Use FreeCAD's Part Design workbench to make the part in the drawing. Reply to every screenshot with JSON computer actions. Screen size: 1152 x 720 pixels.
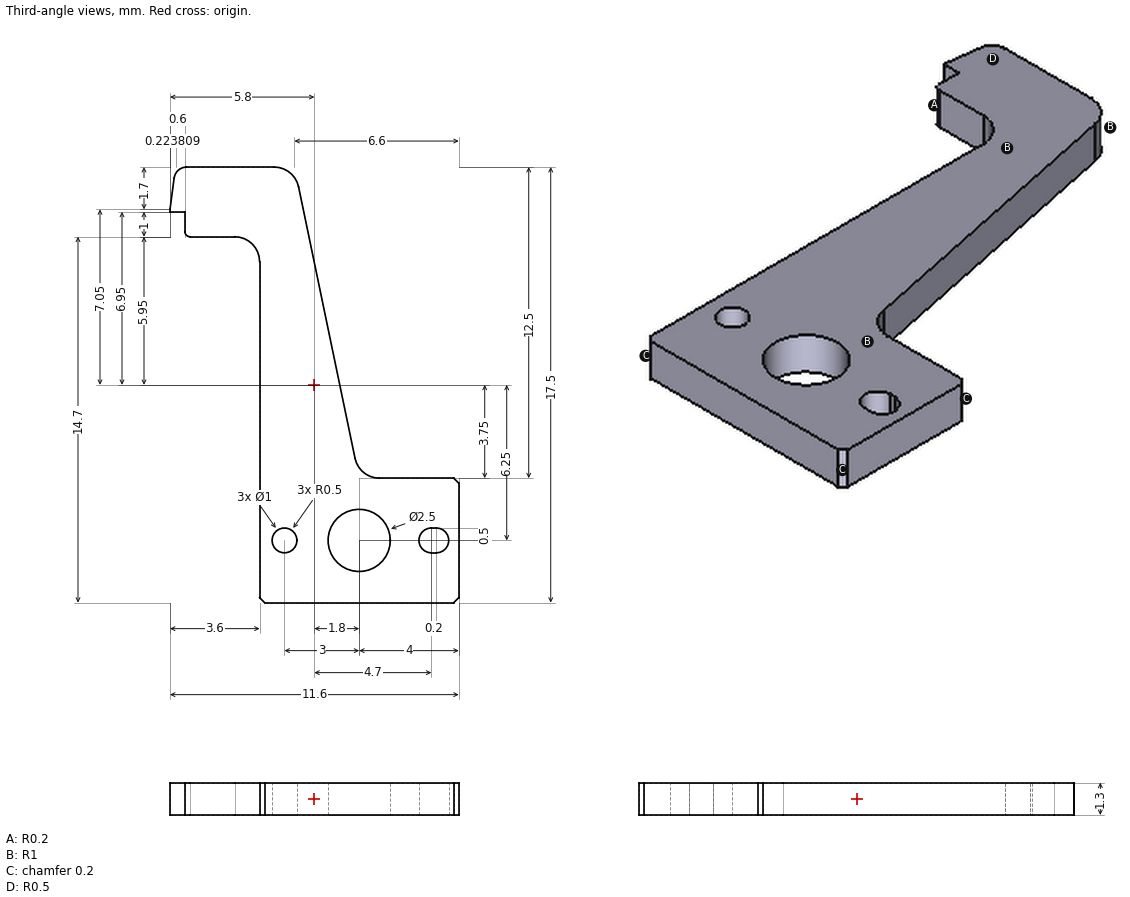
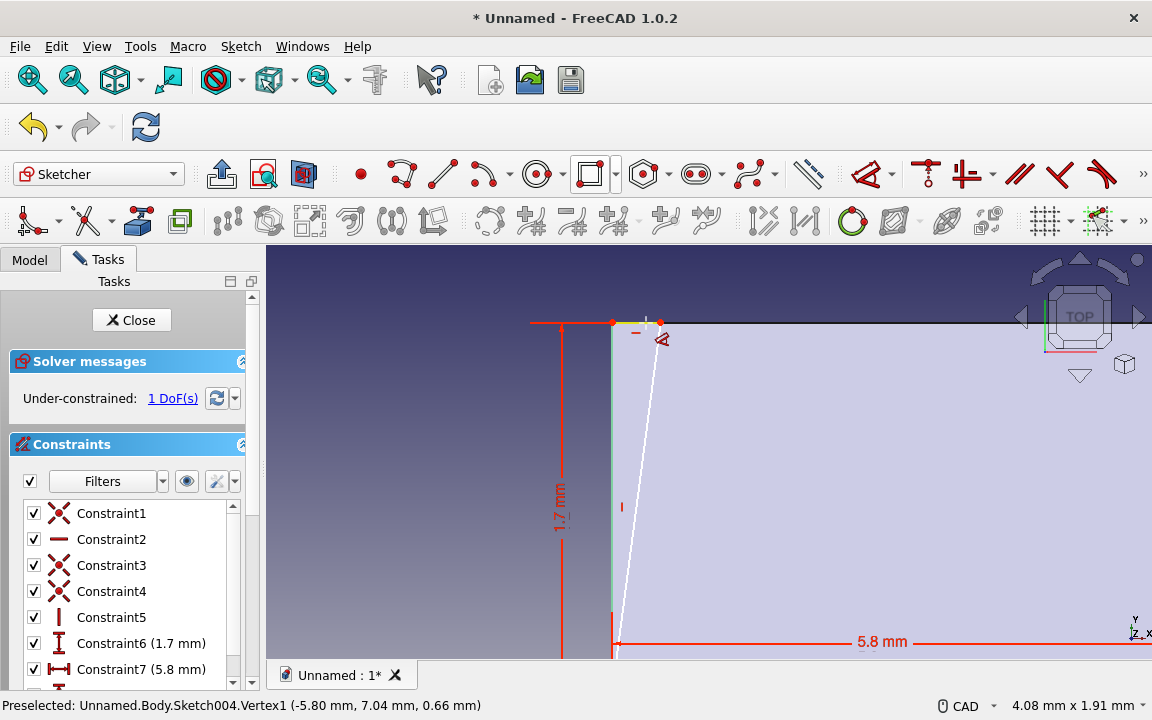
{"action": "left_click", "coordinate": [646, 323]}
{"action": "left_click", "coordinate": [636, 289]}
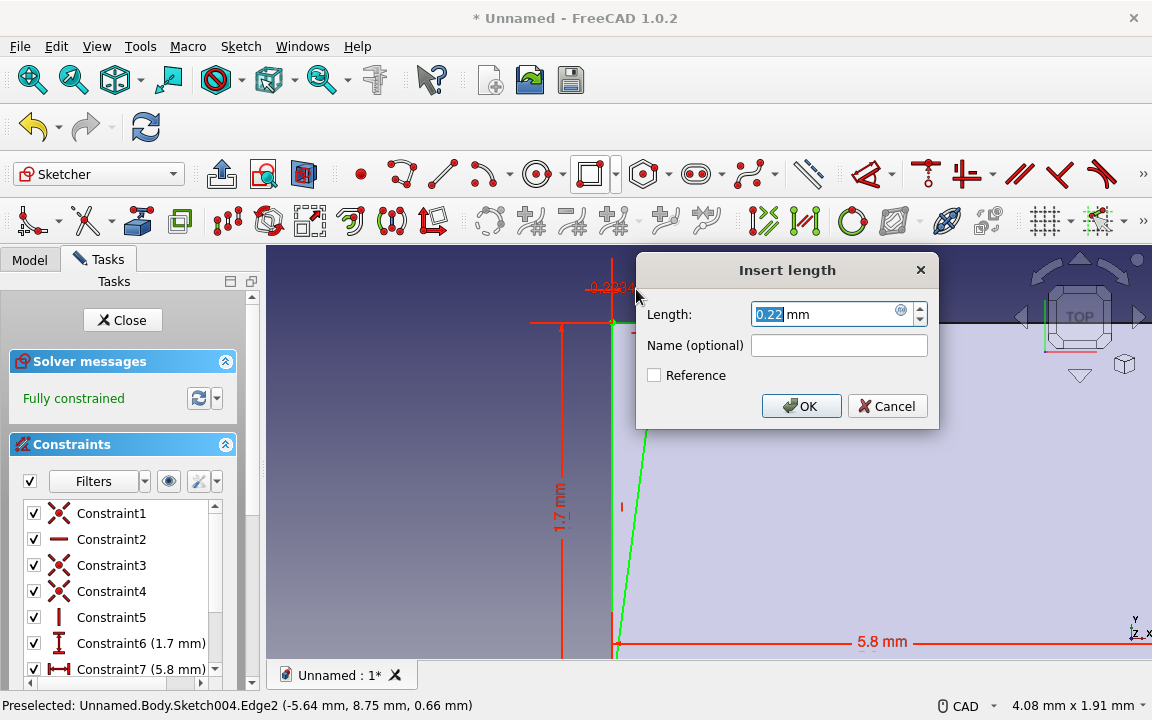
{"action": "type", "text": "0.223809"}
{"action": "key", "text": "Return"}
{"action": "key", "text": "Escape"}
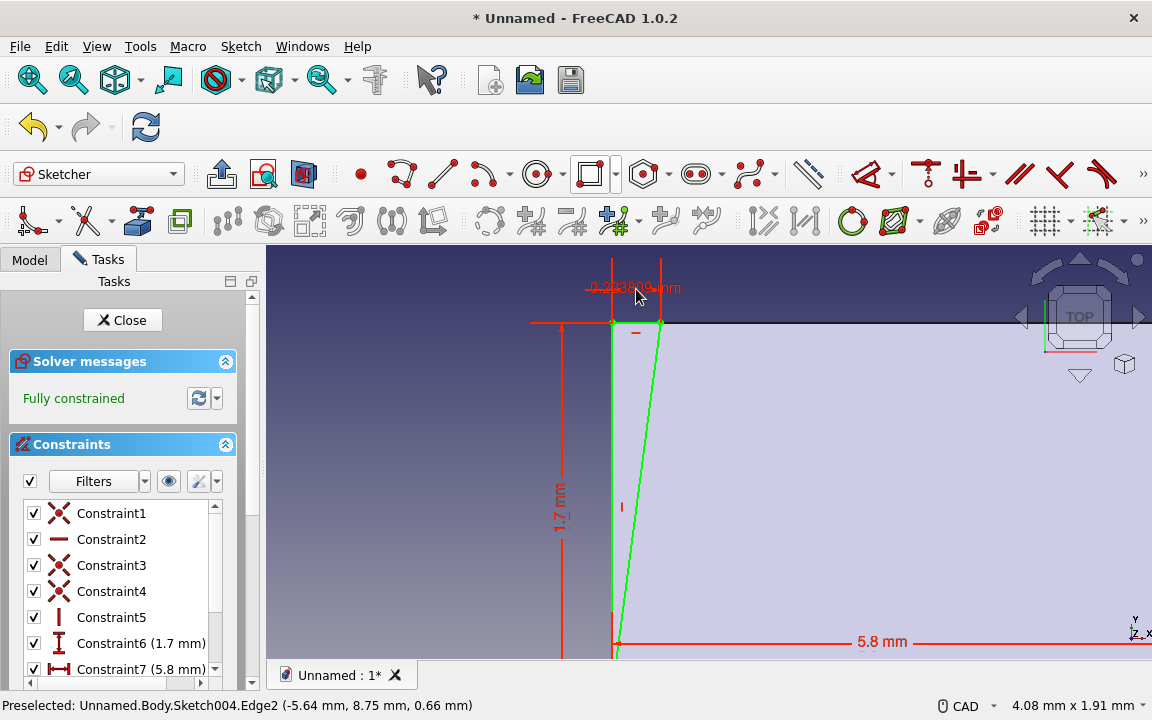
{"action": "left_click", "coordinate": [123, 320]}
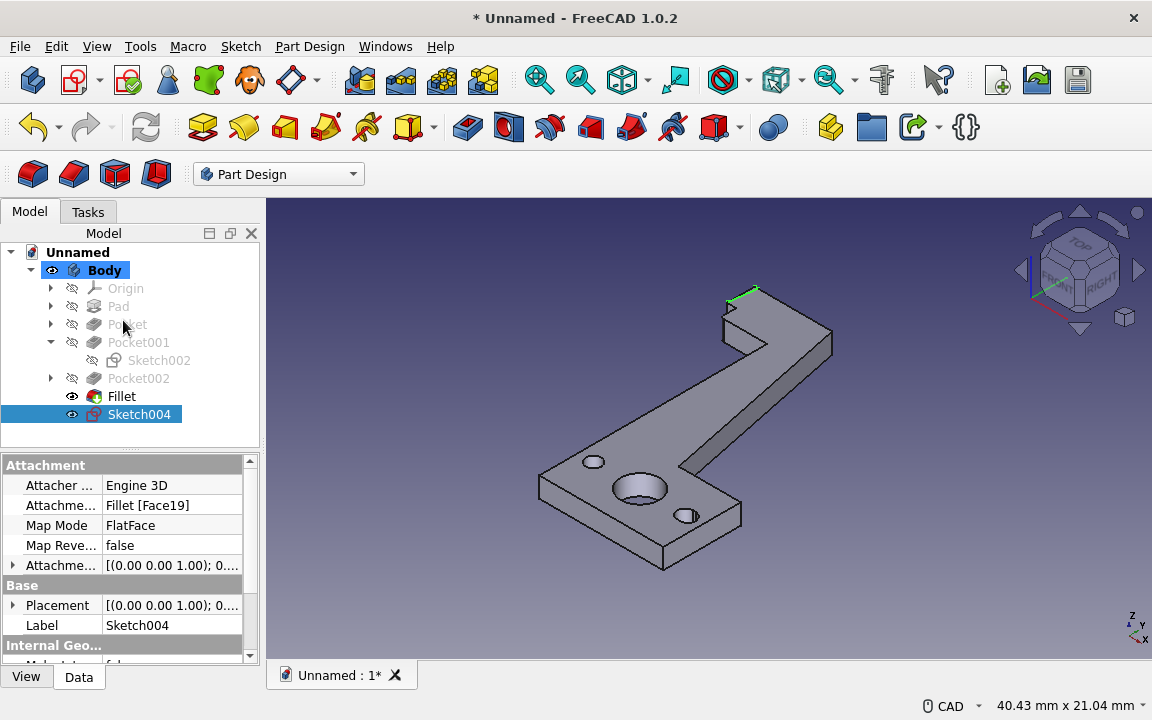
{"action": "left_click", "coordinate": [468, 128]}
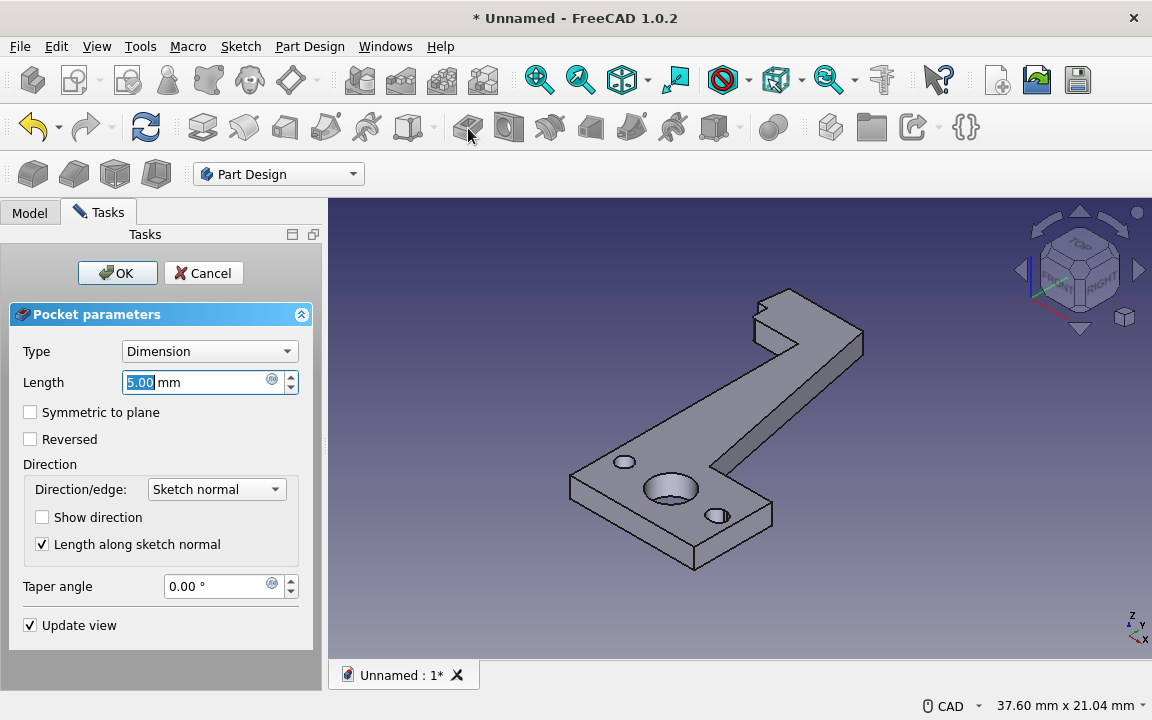
{"action": "left_click", "coordinate": [210, 352]}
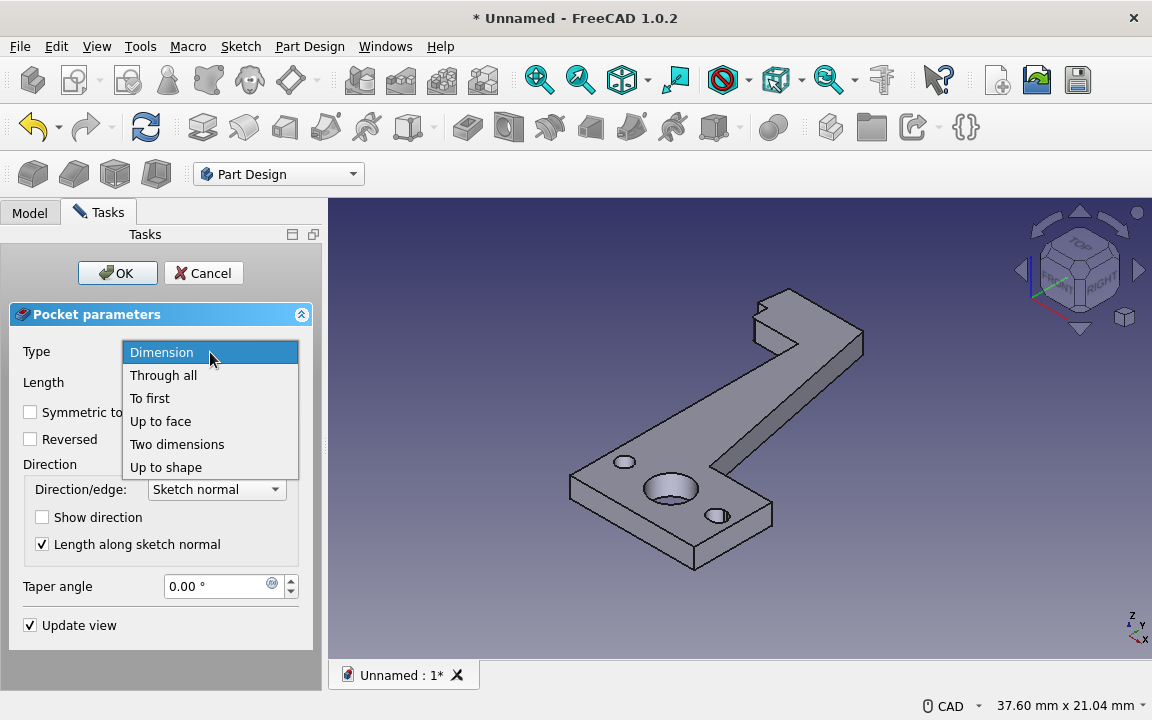
{"action": "left_click", "coordinate": [208, 376]}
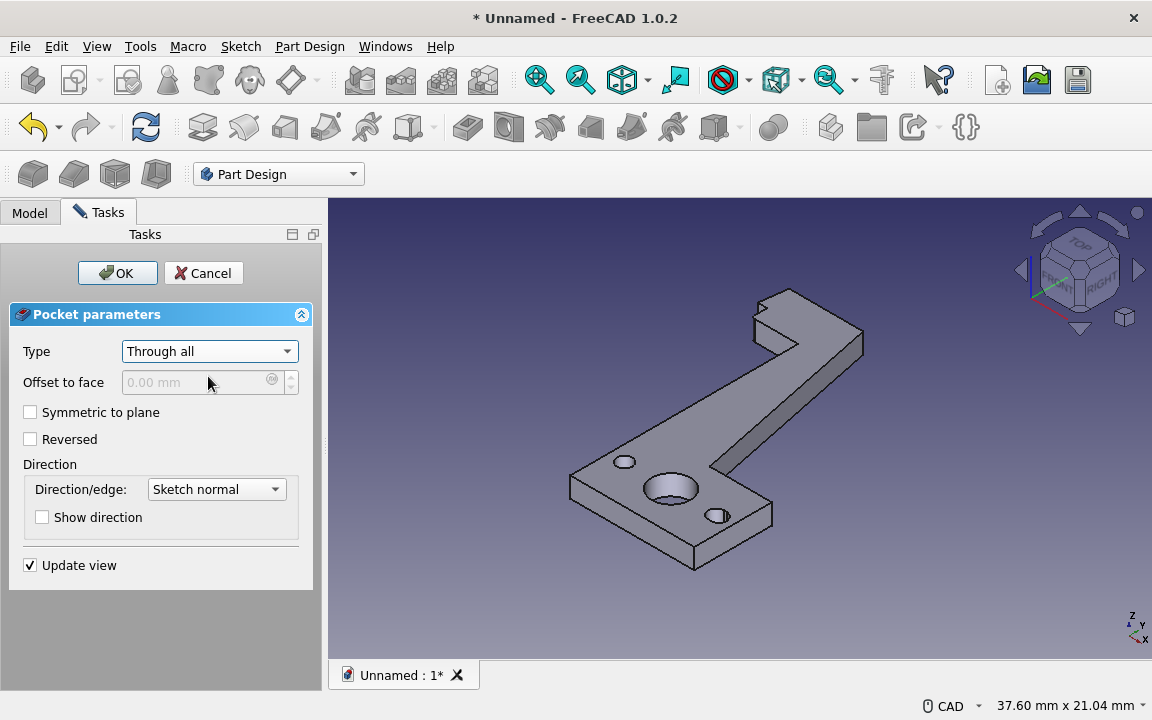
{"action": "left_click", "coordinate": [118, 273]}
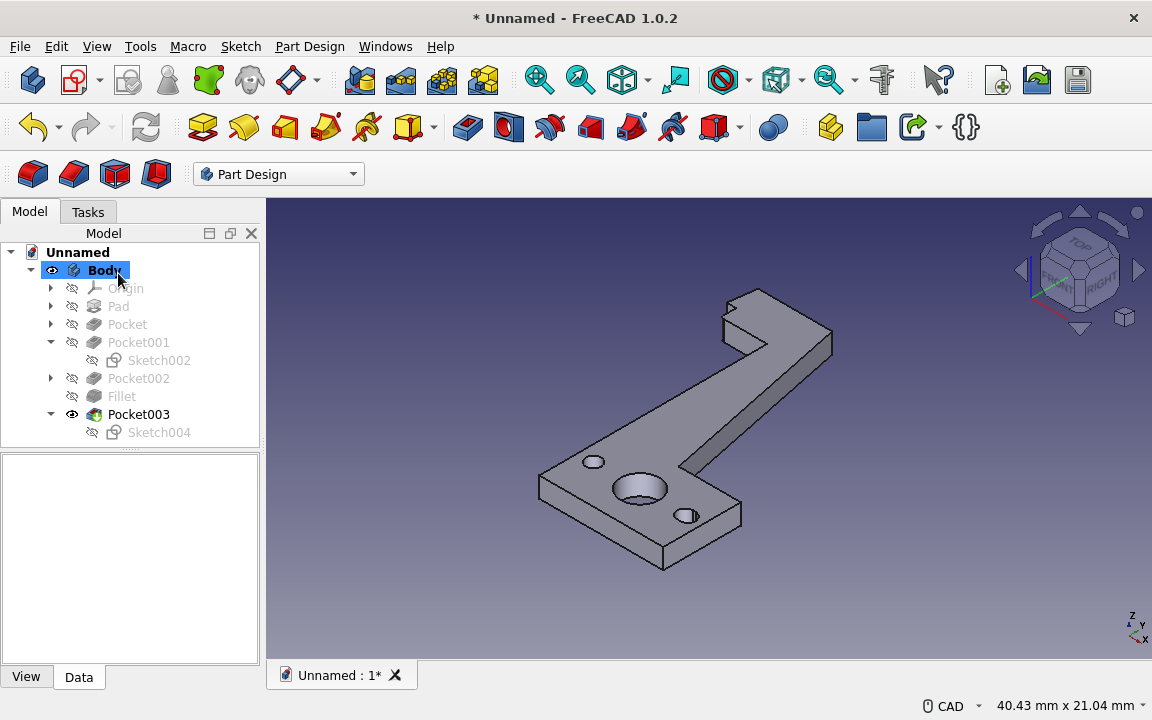
{"action": "key", "text": "2"}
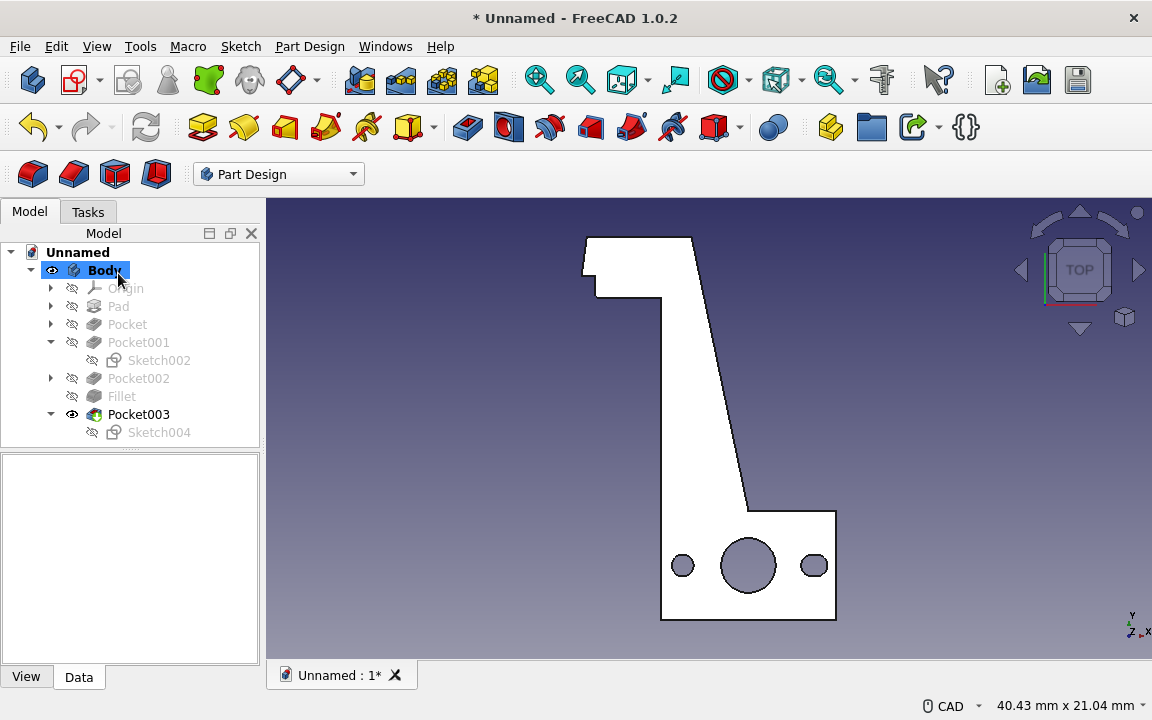
{"action": "key", "text": "0"}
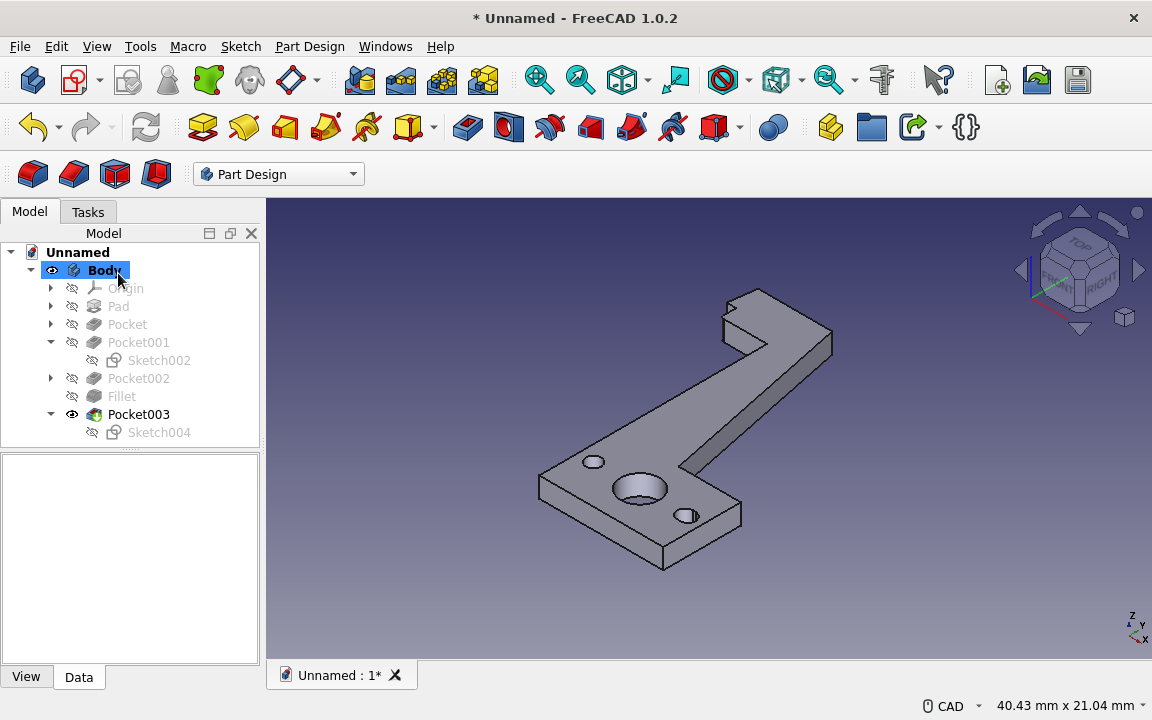
{"action": "key", "text": "1"}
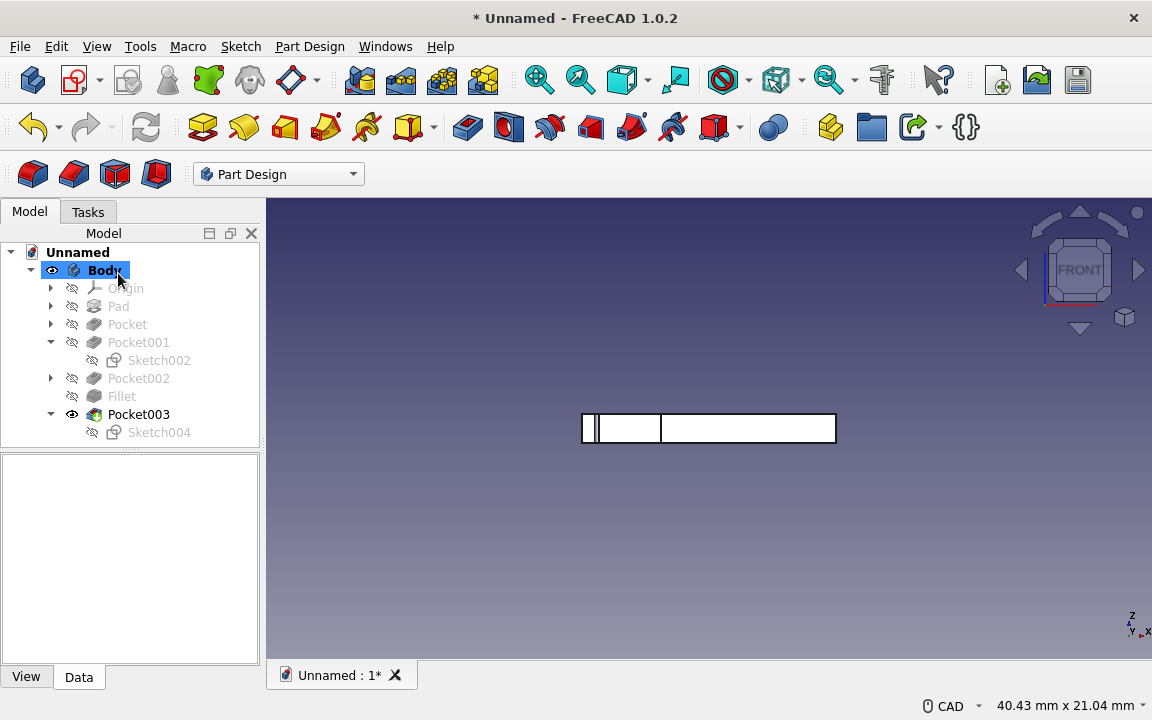
{"action": "left_click", "coordinate": [540, 80]}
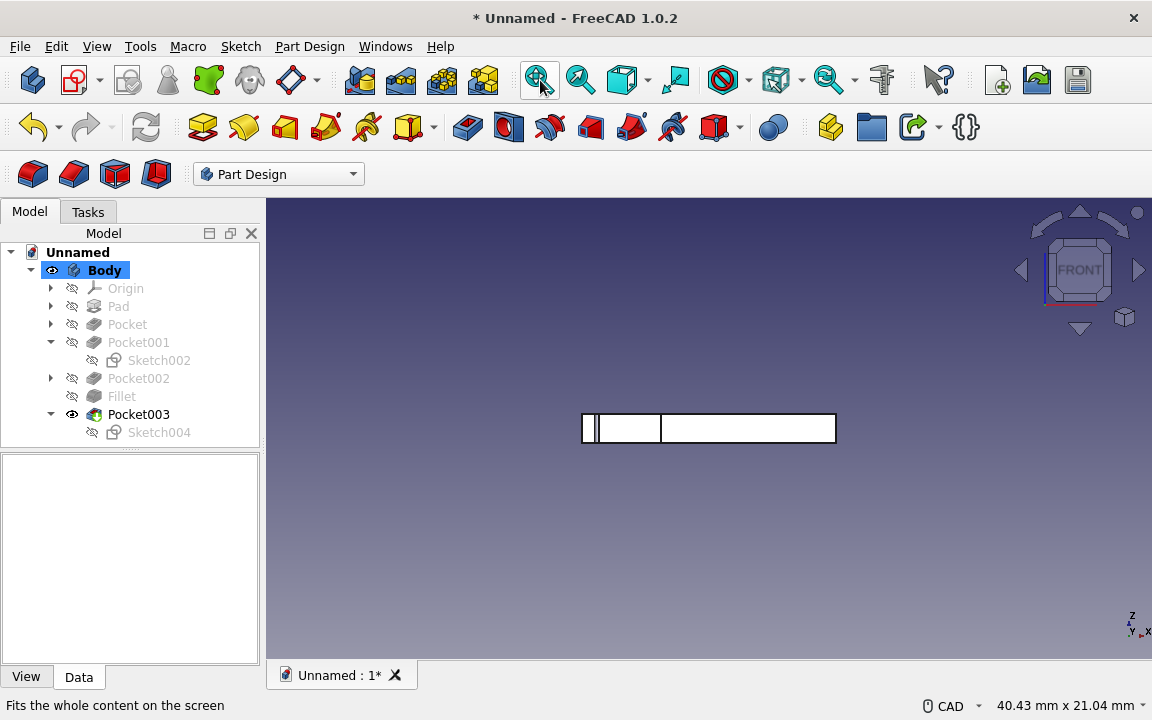
{"action": "key", "text": "3"}